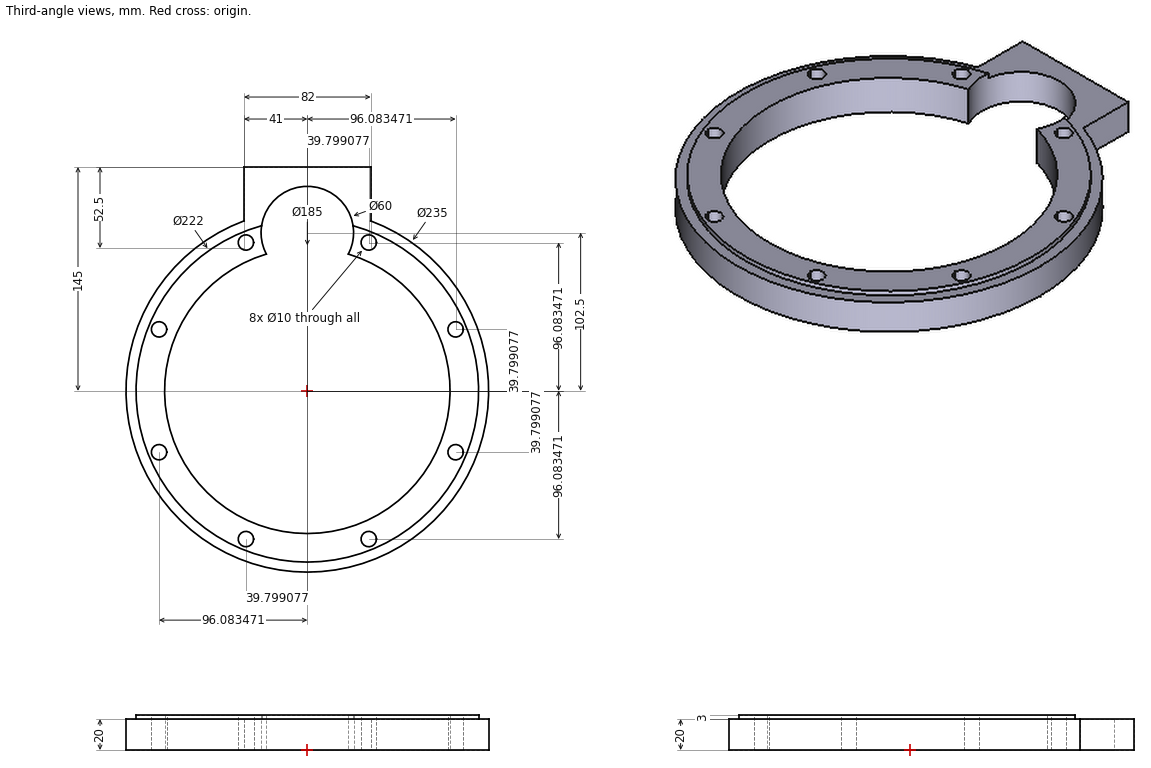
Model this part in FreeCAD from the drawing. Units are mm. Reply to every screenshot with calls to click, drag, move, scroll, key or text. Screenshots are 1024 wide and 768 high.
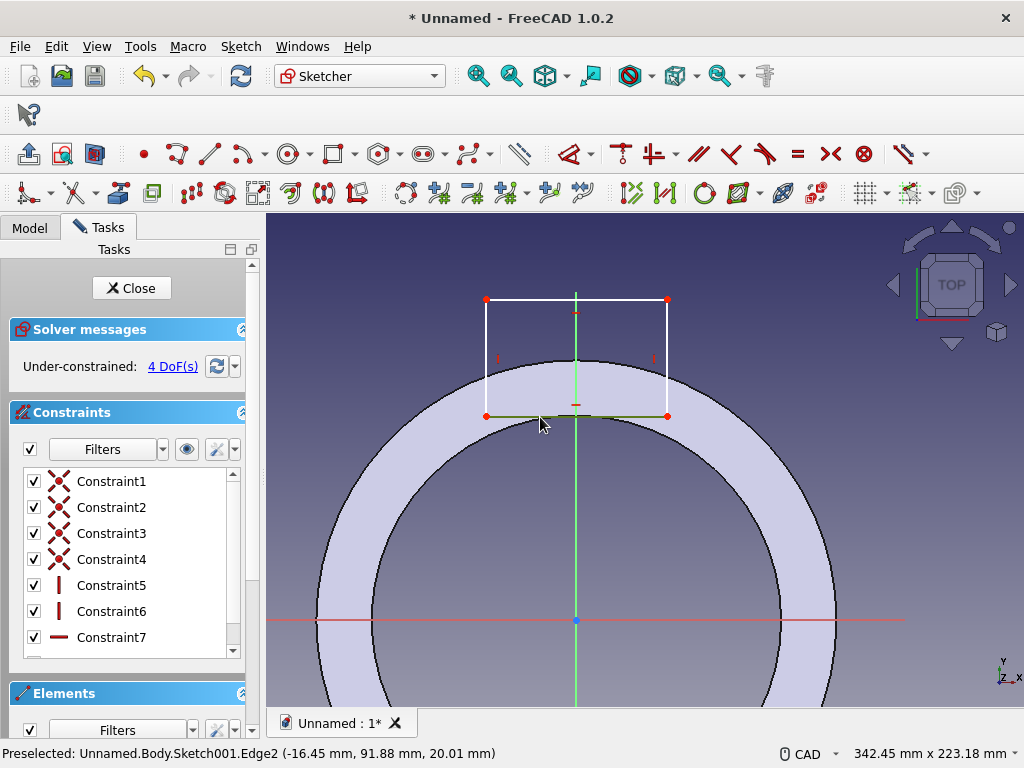
key(l)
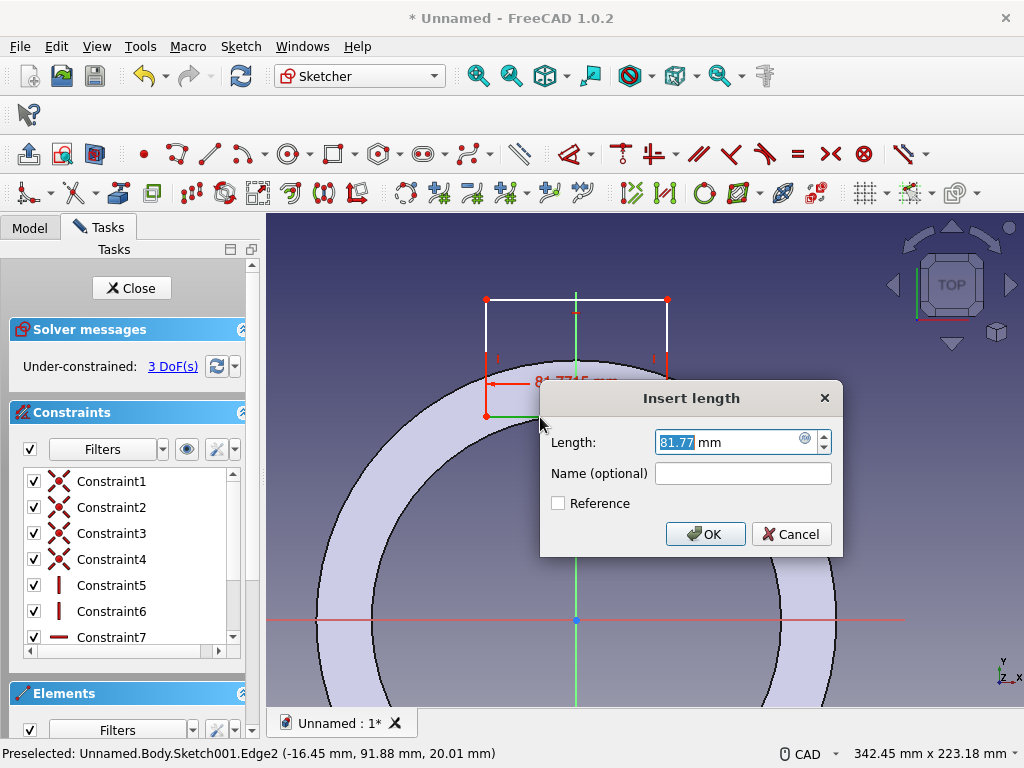
text(82)
key(Return)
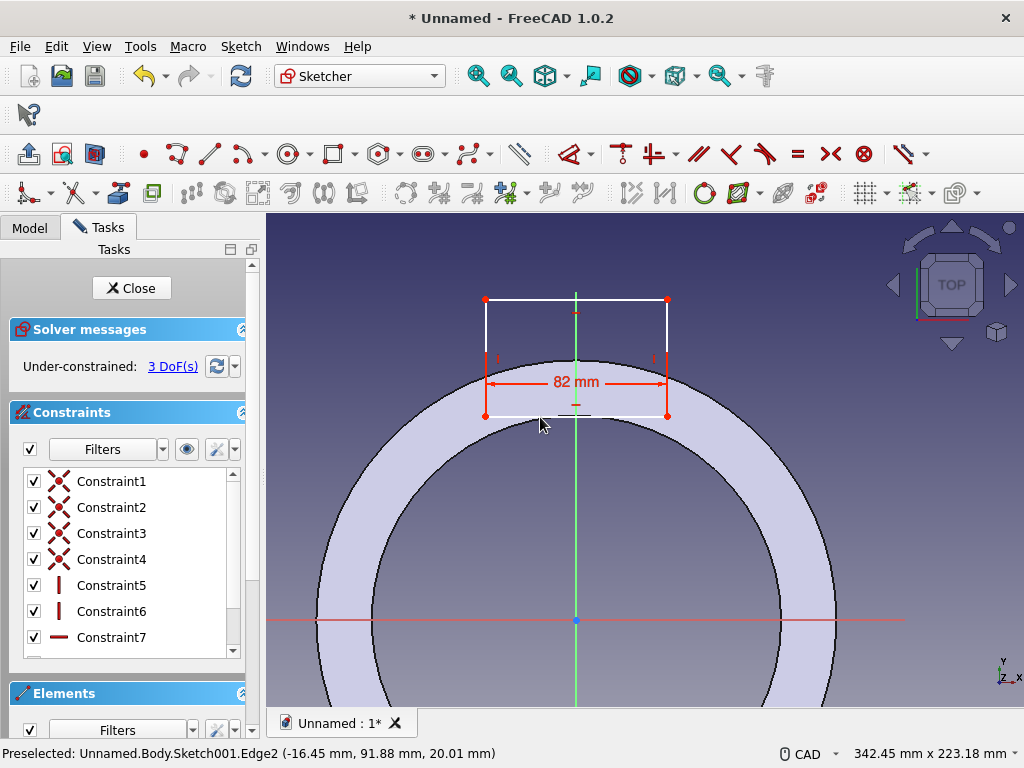
click(486, 300)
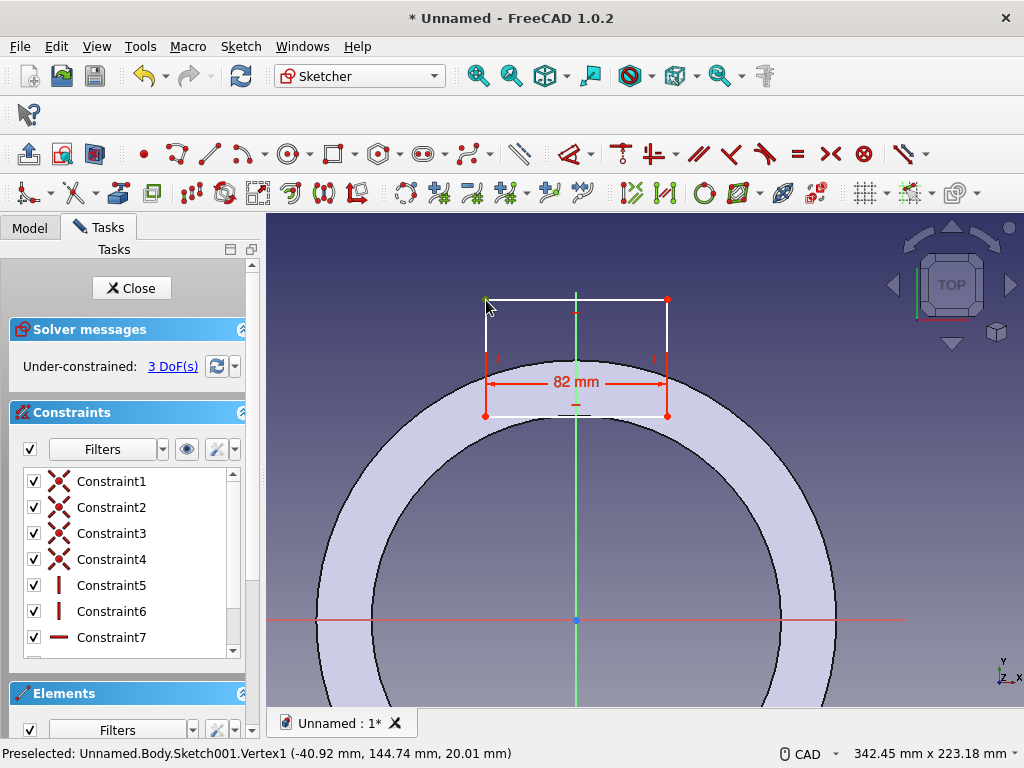
click(590, 154)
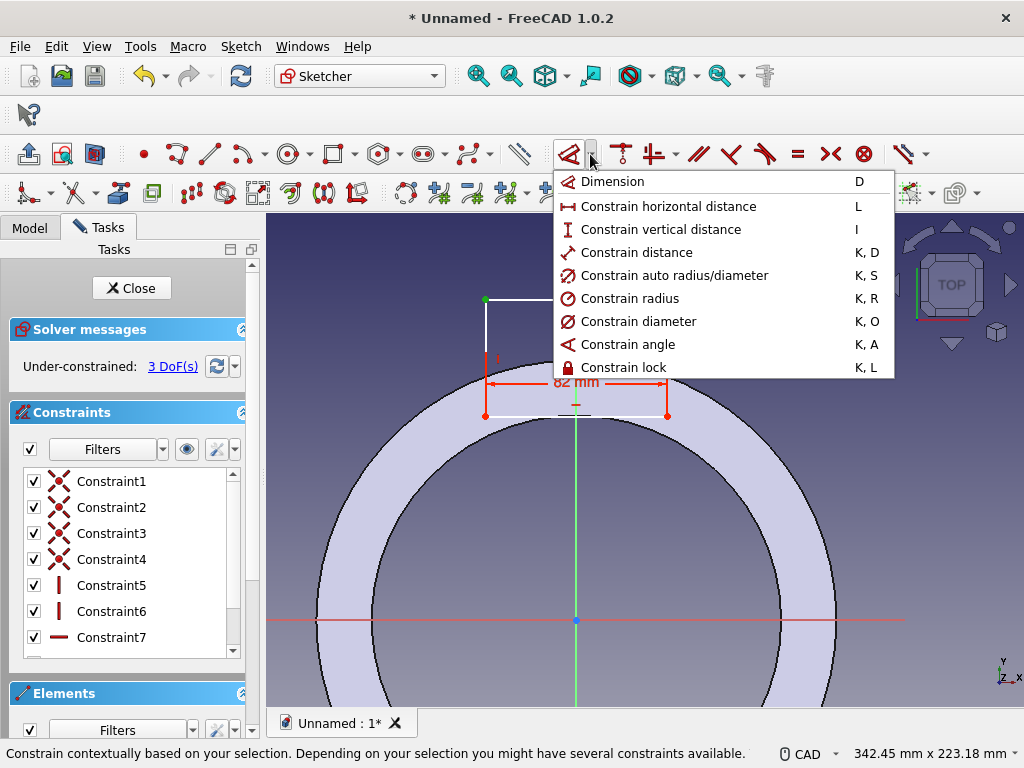
click(724, 206)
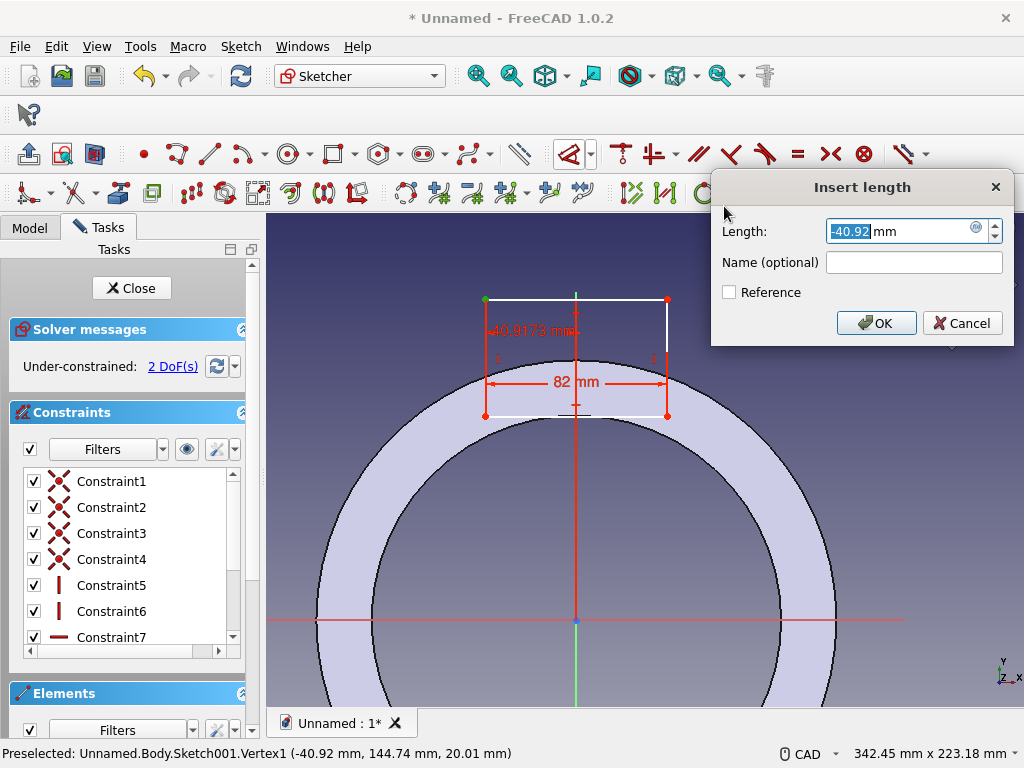
text(-41)
key(Return)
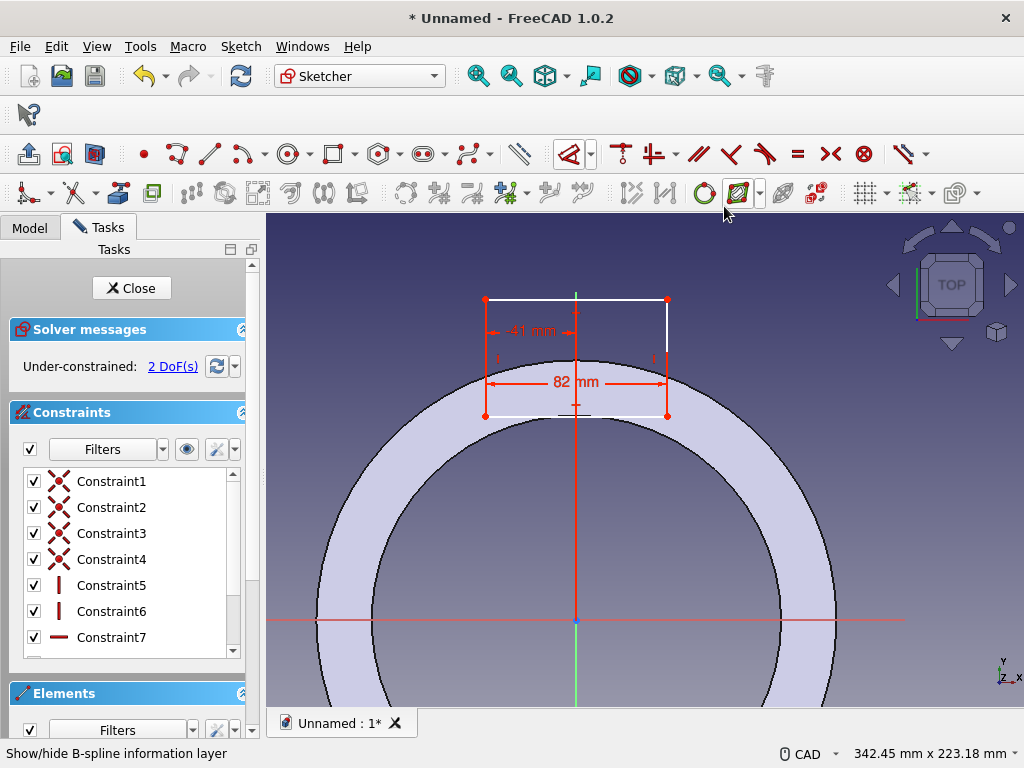
click(486, 335)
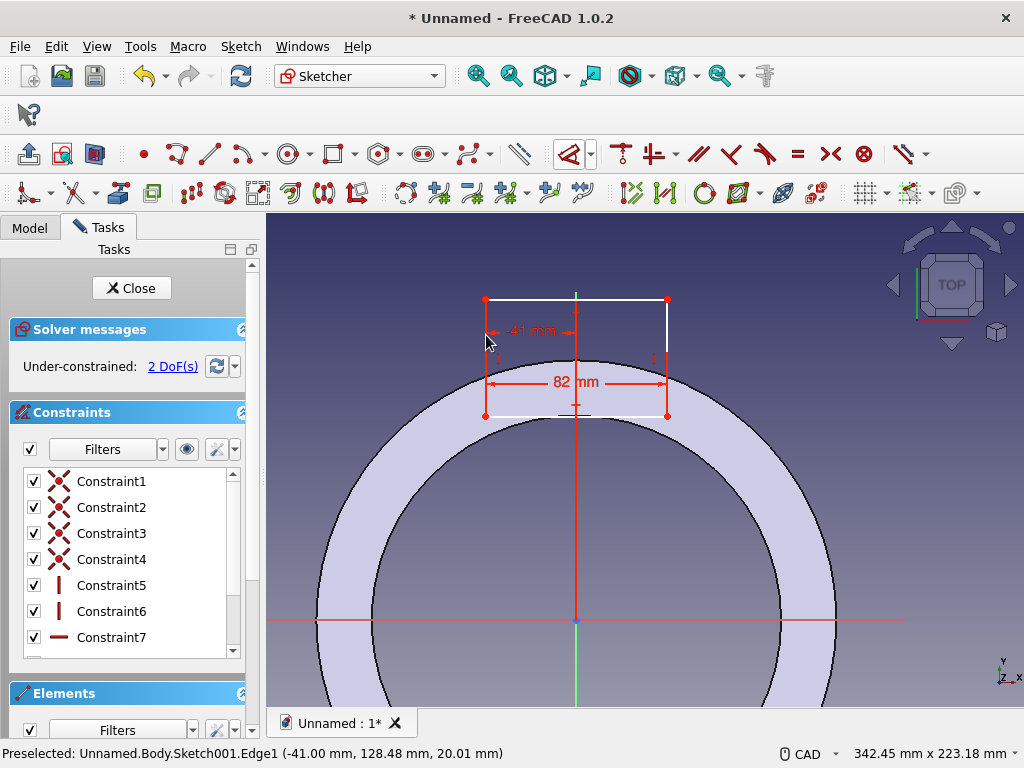
key(i)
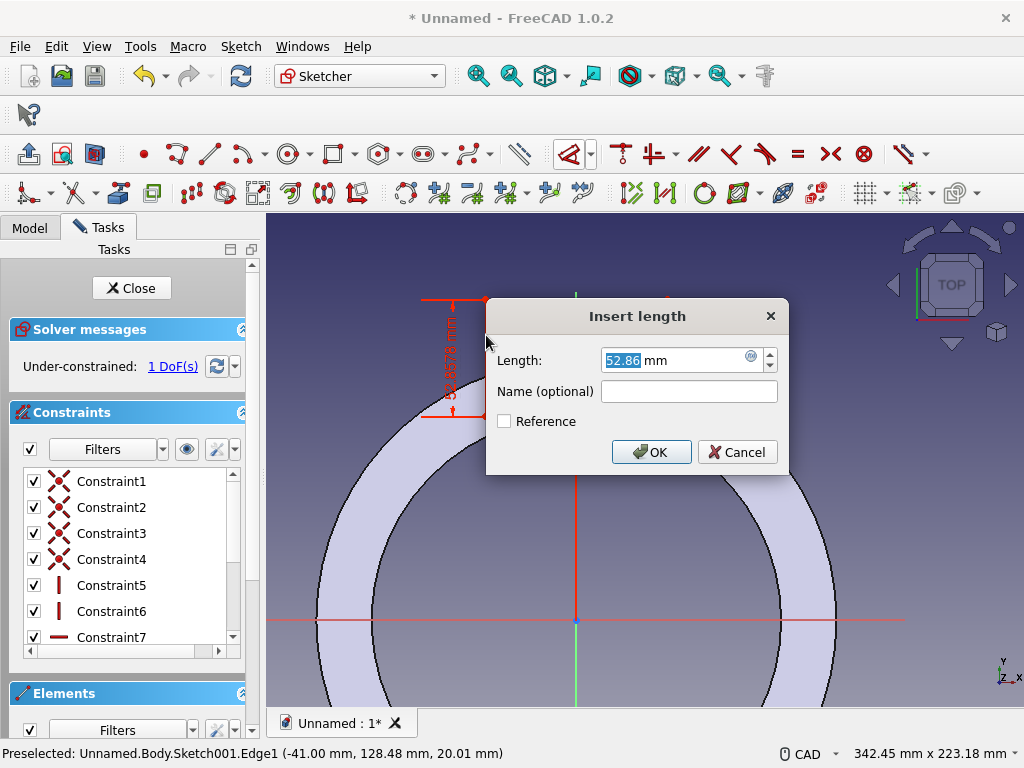
text(52.5)
key(Return)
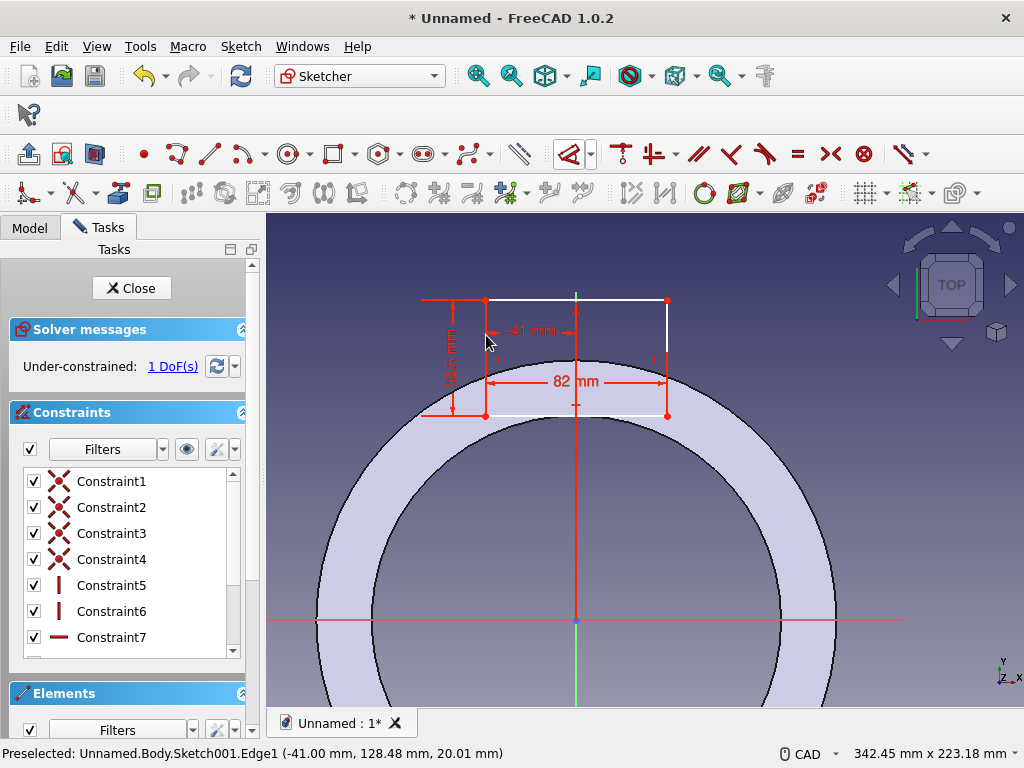
click(486, 300)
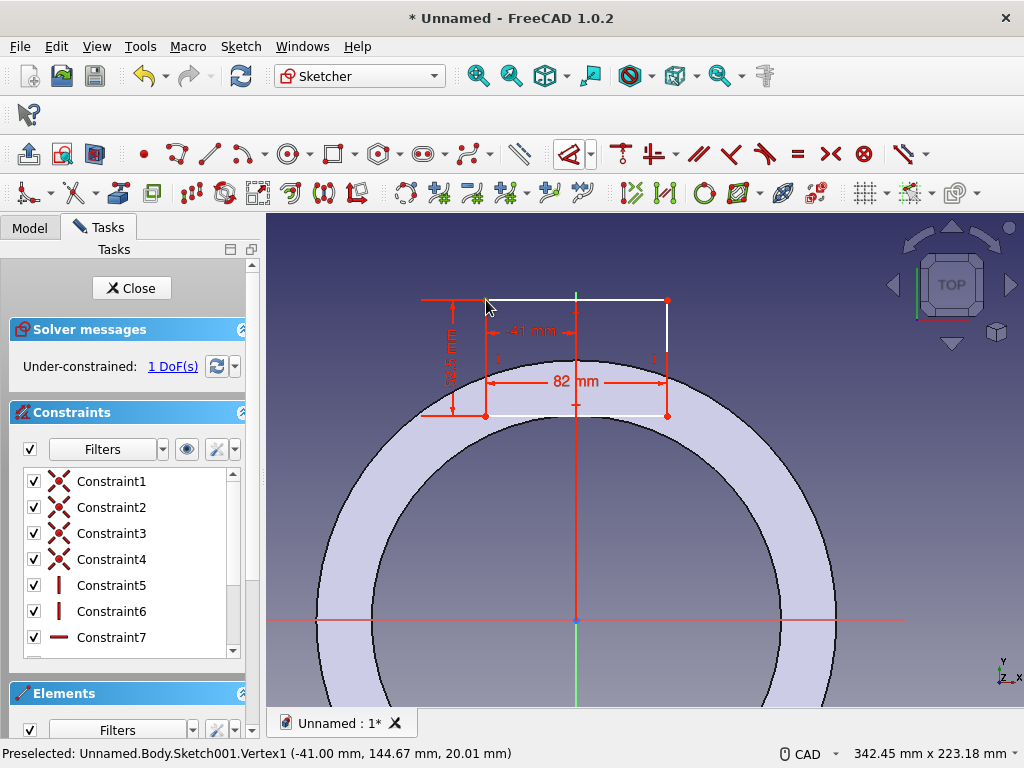
key(i)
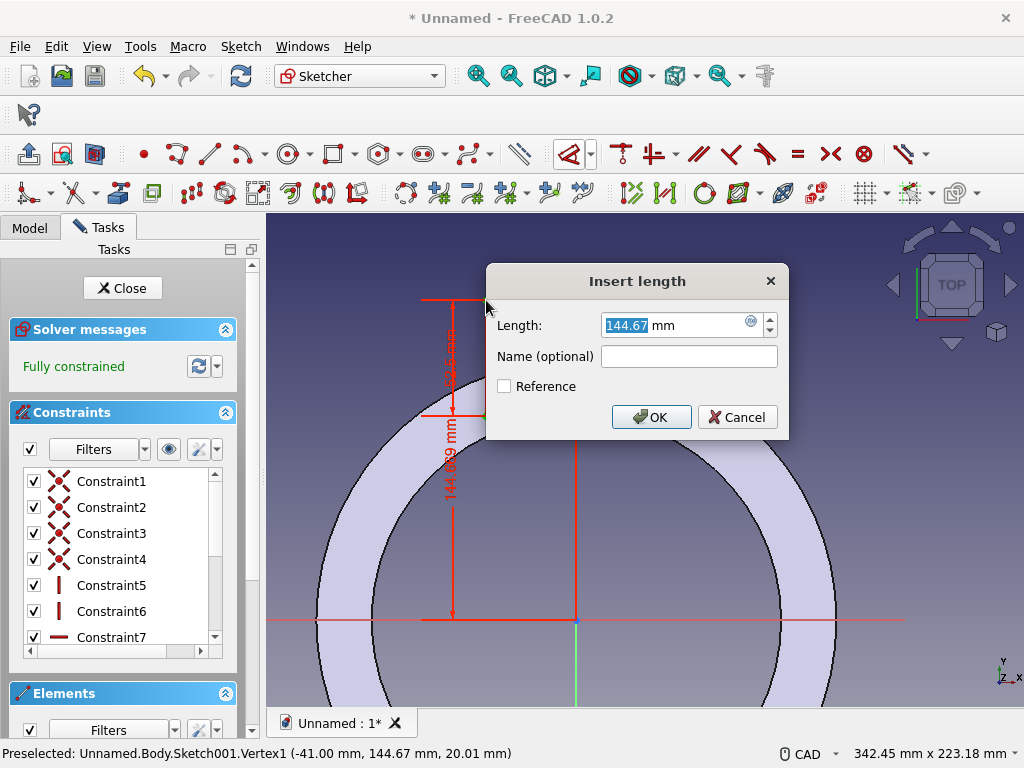
text(145)
key(Return)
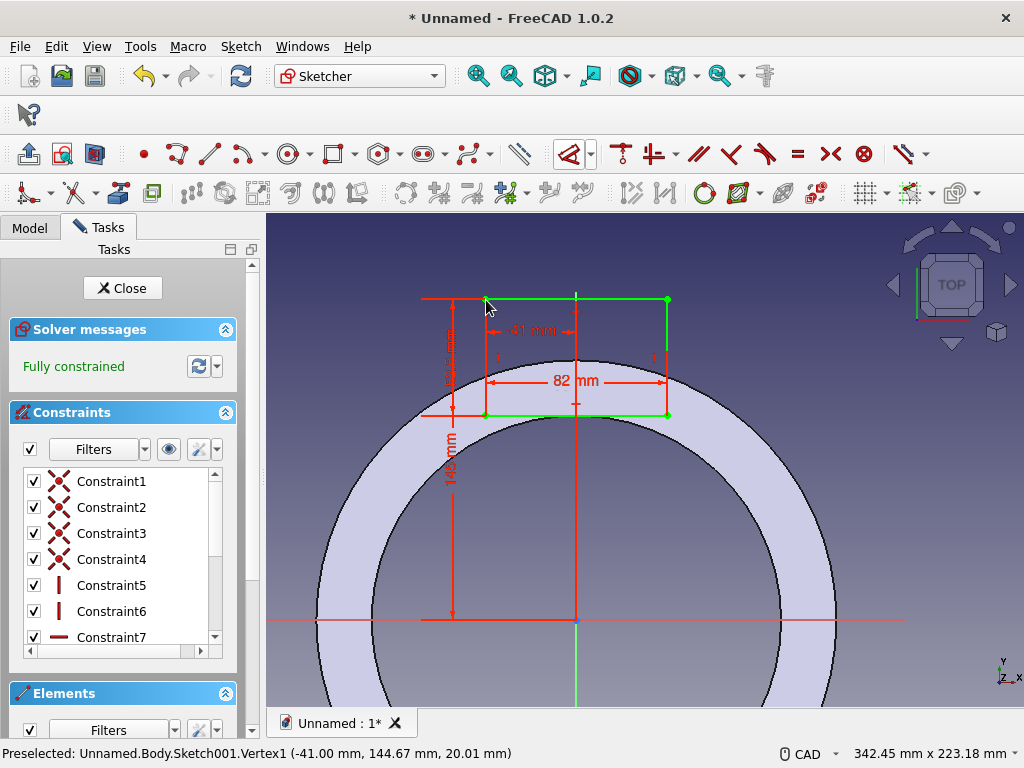
click(123, 288)